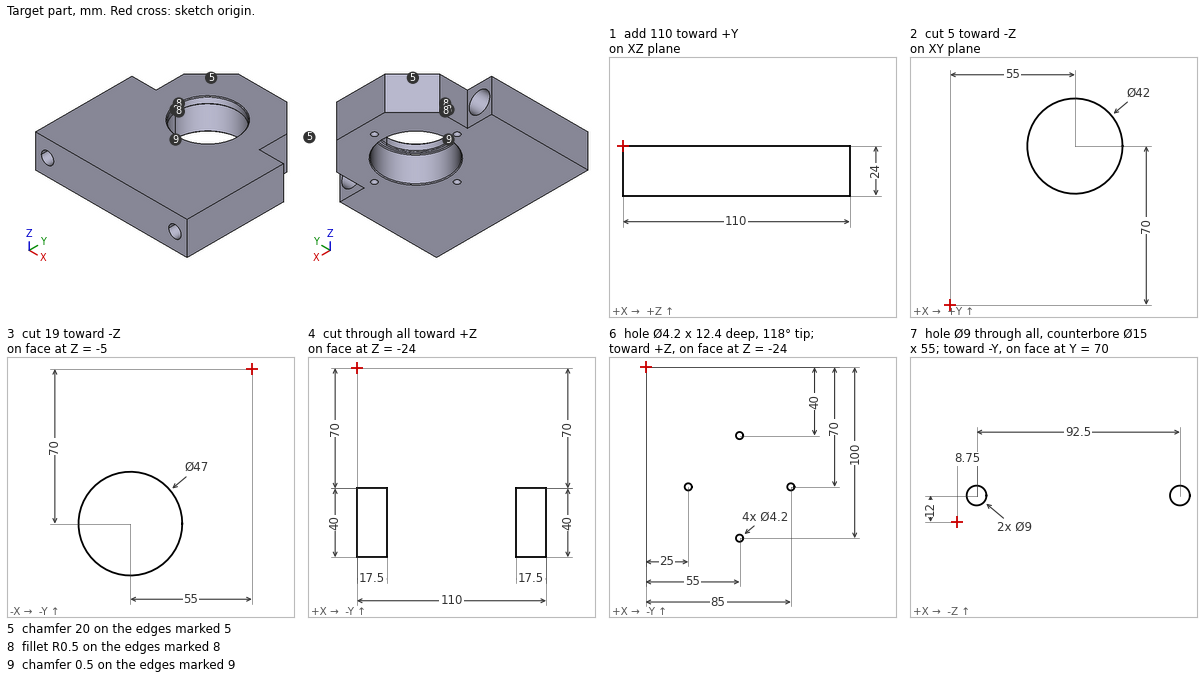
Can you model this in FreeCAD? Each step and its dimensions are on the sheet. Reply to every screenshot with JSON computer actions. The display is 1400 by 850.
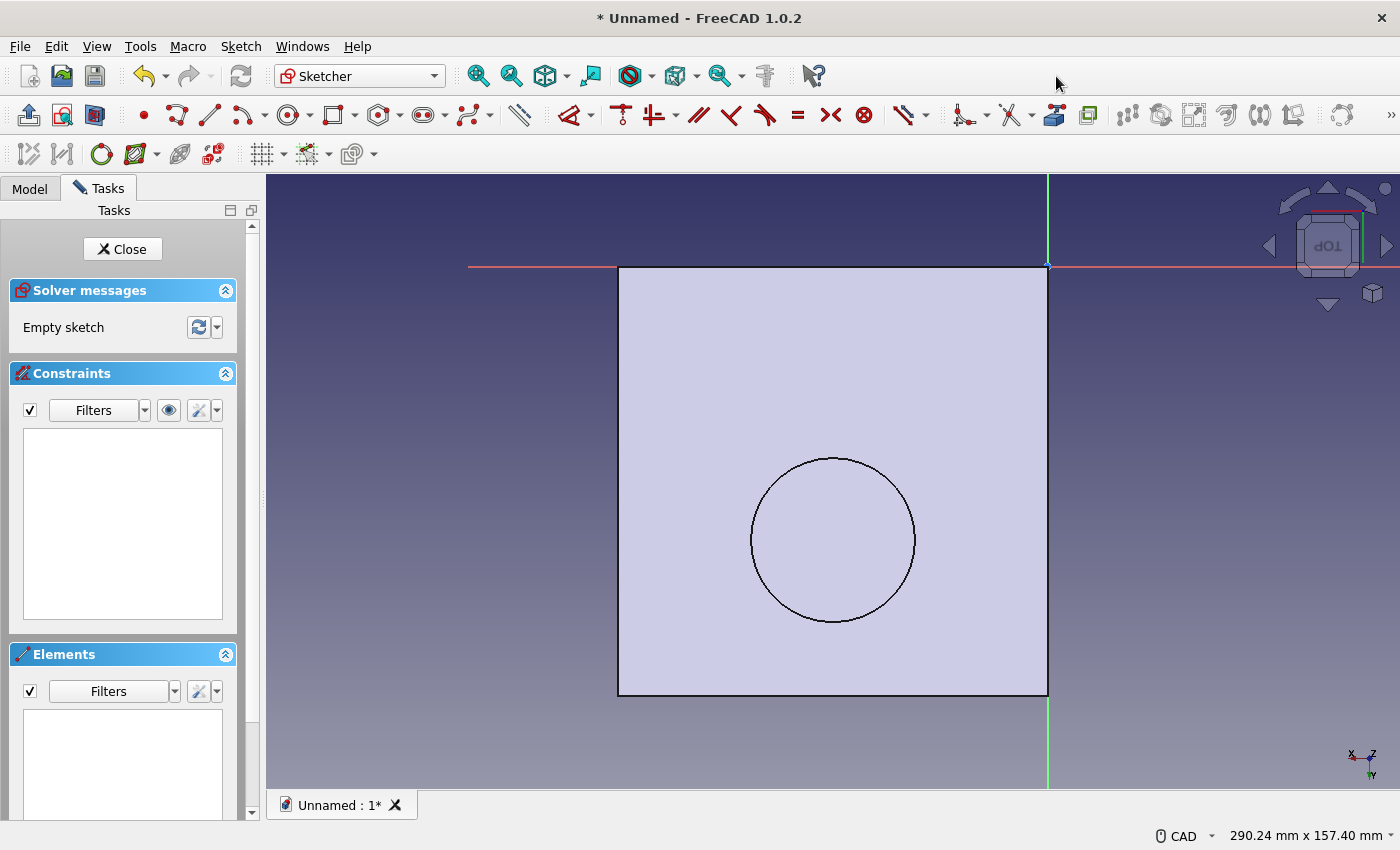
{"action": "left_click", "coordinate": [288, 116]}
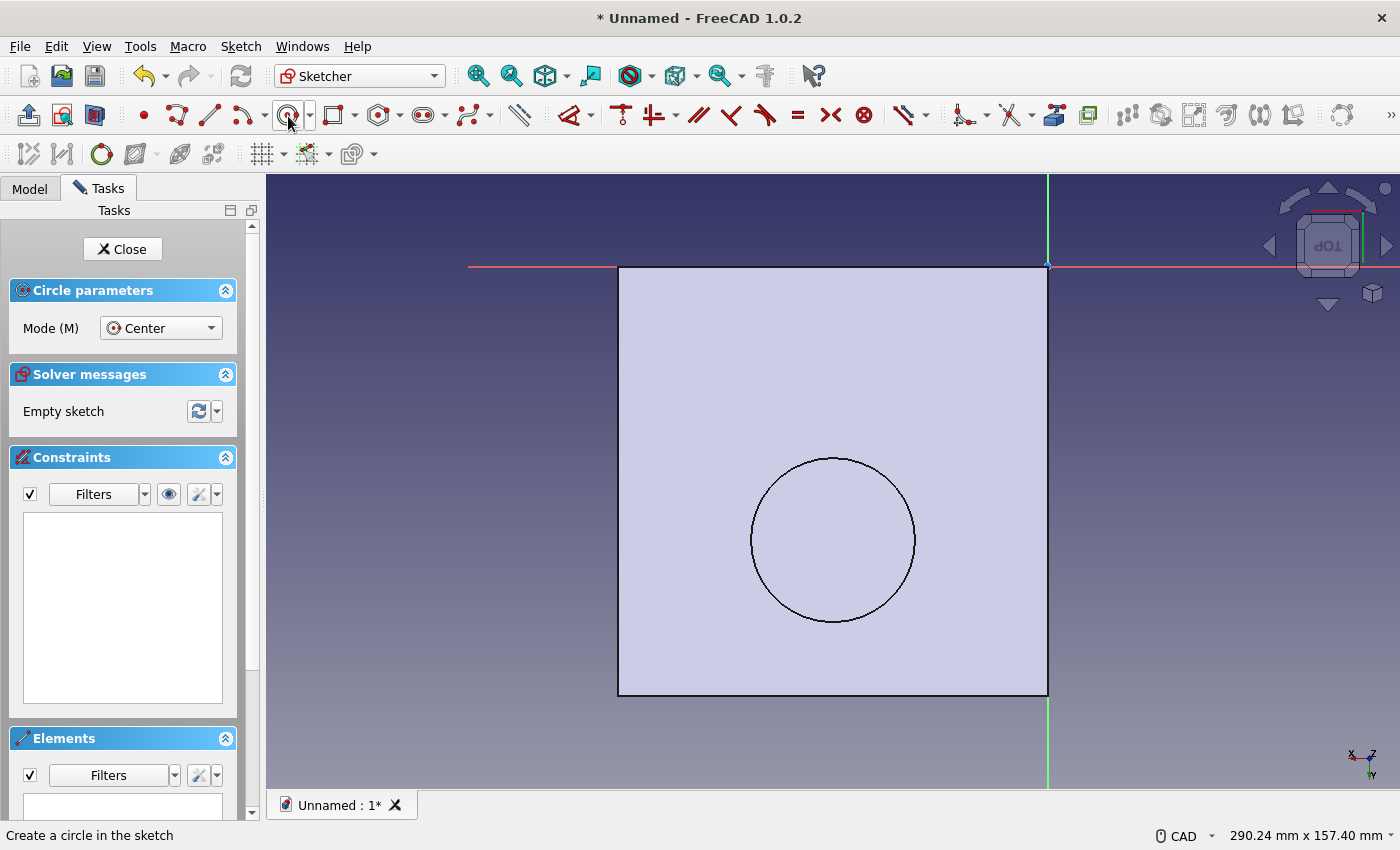
{"action": "left_click", "coordinate": [833, 540]}
{"action": "mouse_move", "coordinate": [898, 475]}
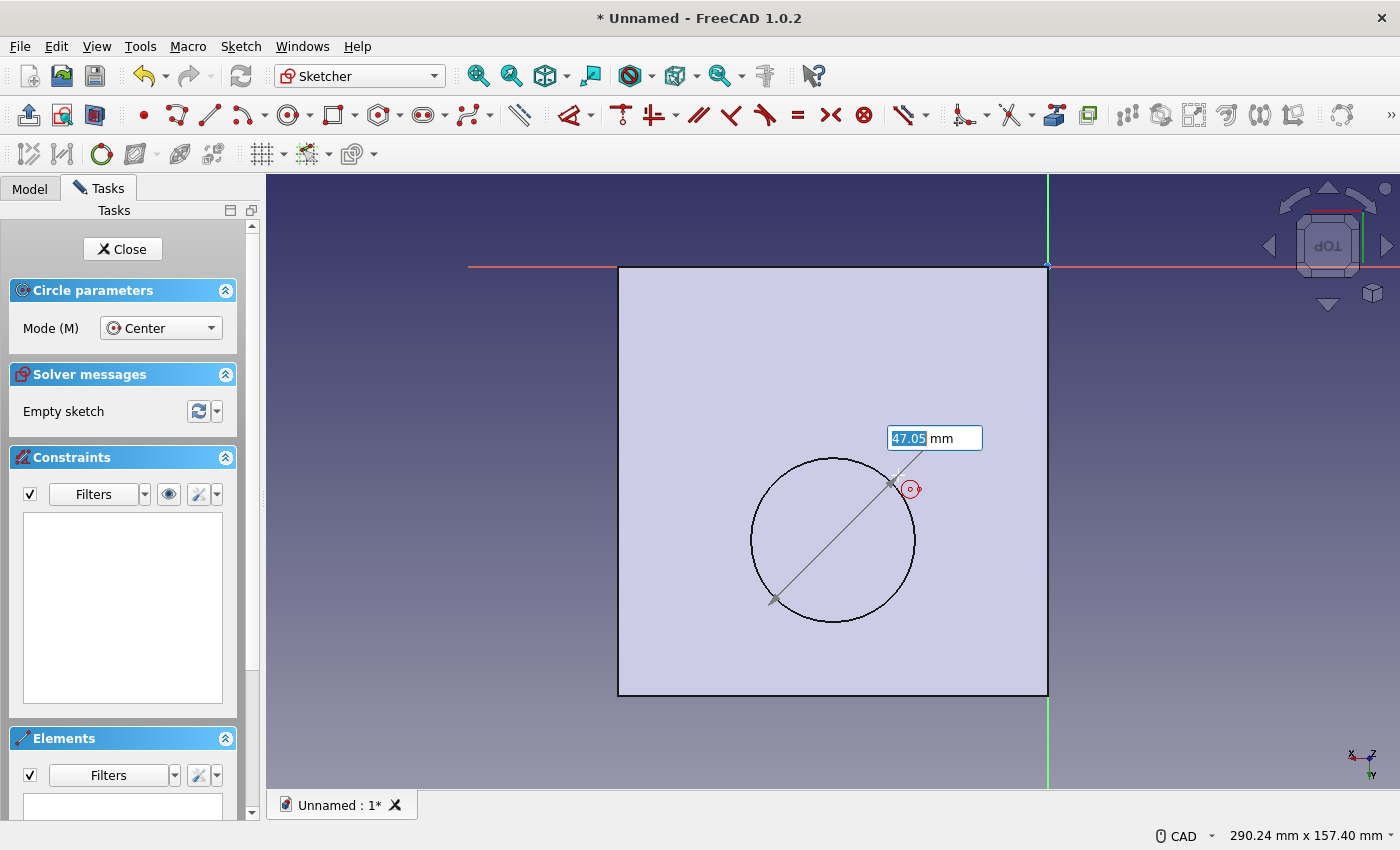
{"action": "type", "text": "47"}
{"action": "key", "text": "Return"}
{"action": "key", "text": "Escape"}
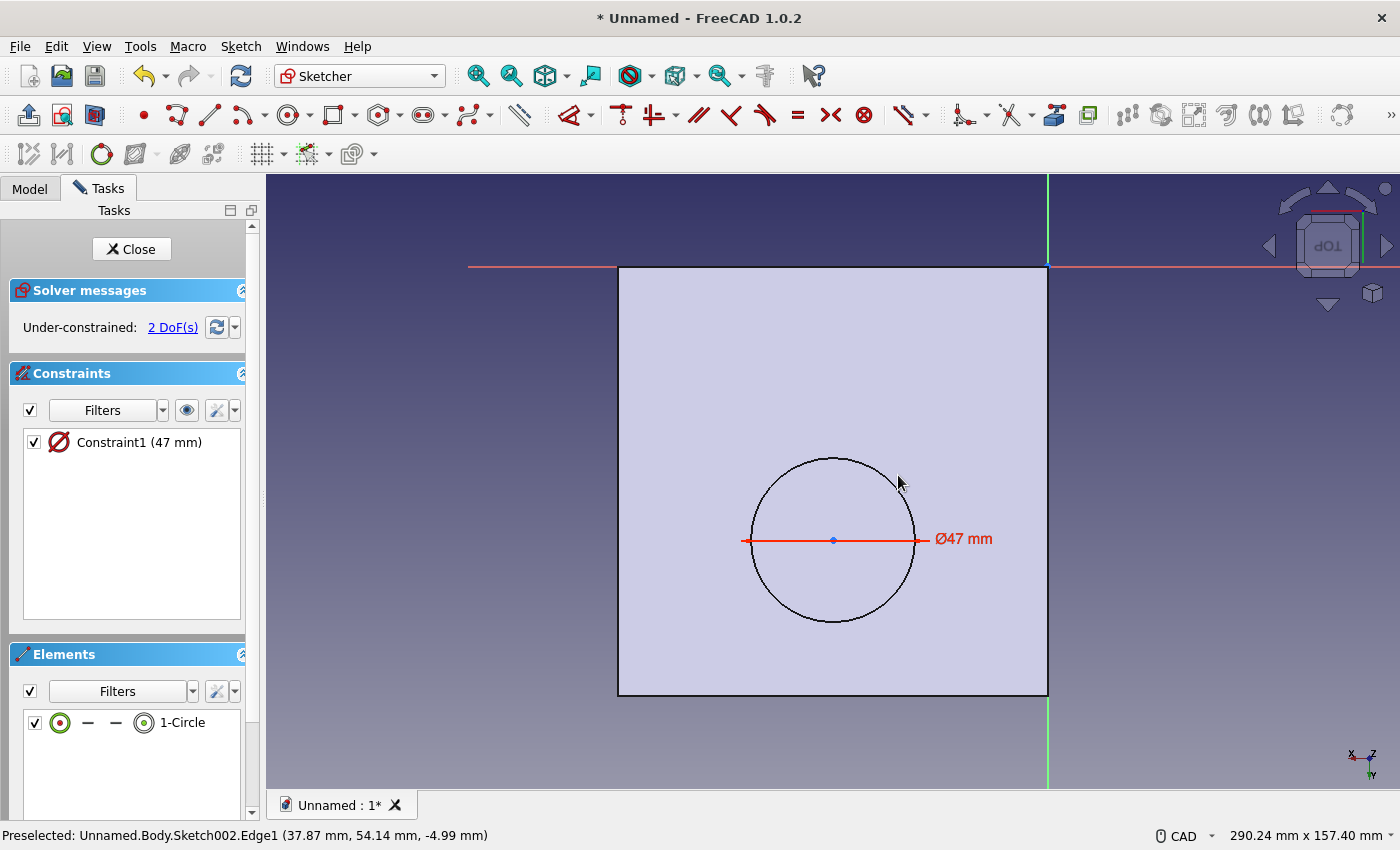
{"action": "left_click", "coordinate": [568, 116]}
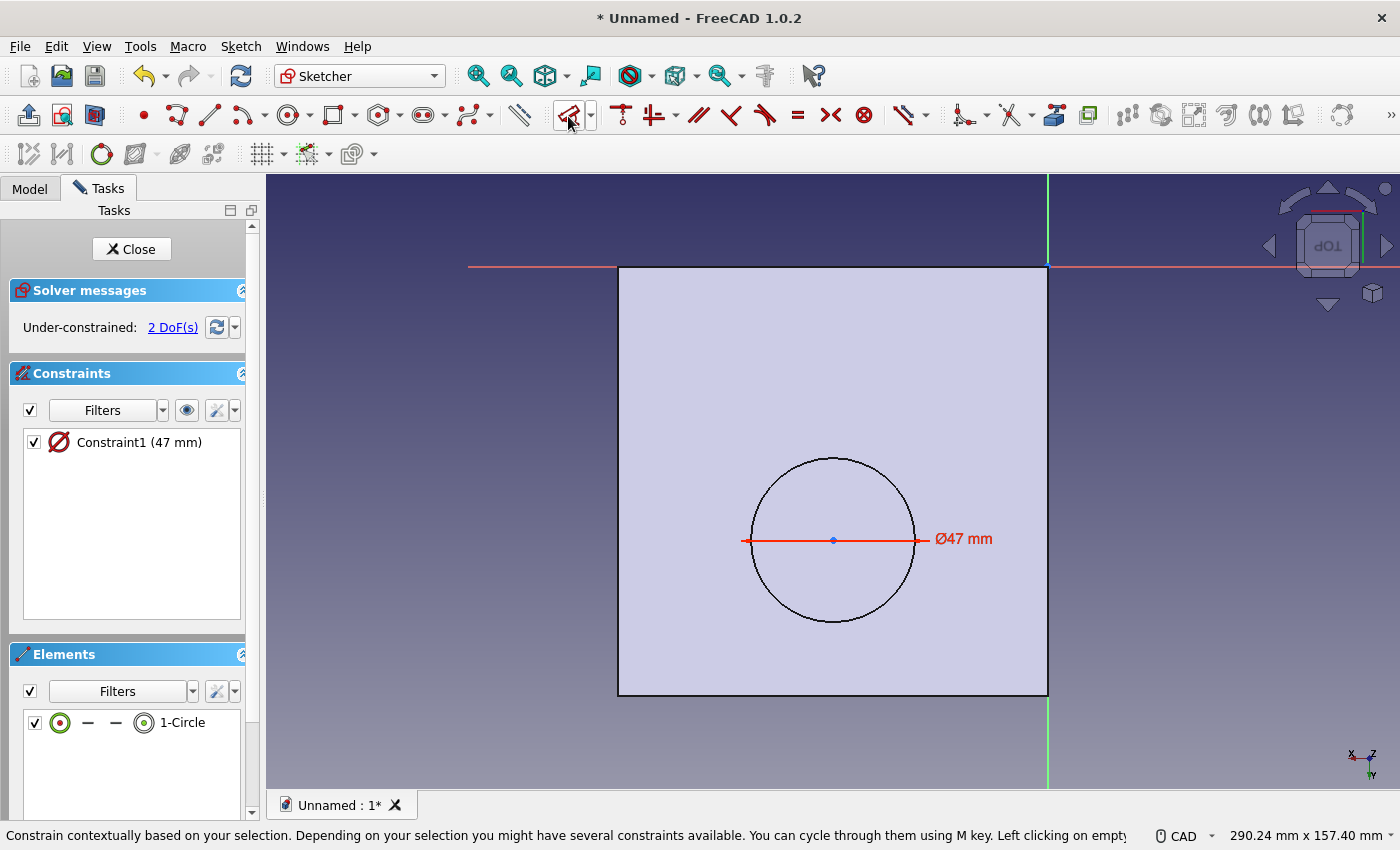
{"action": "left_click", "coordinate": [833, 541]}
{"action": "left_click", "coordinate": [940, 233]}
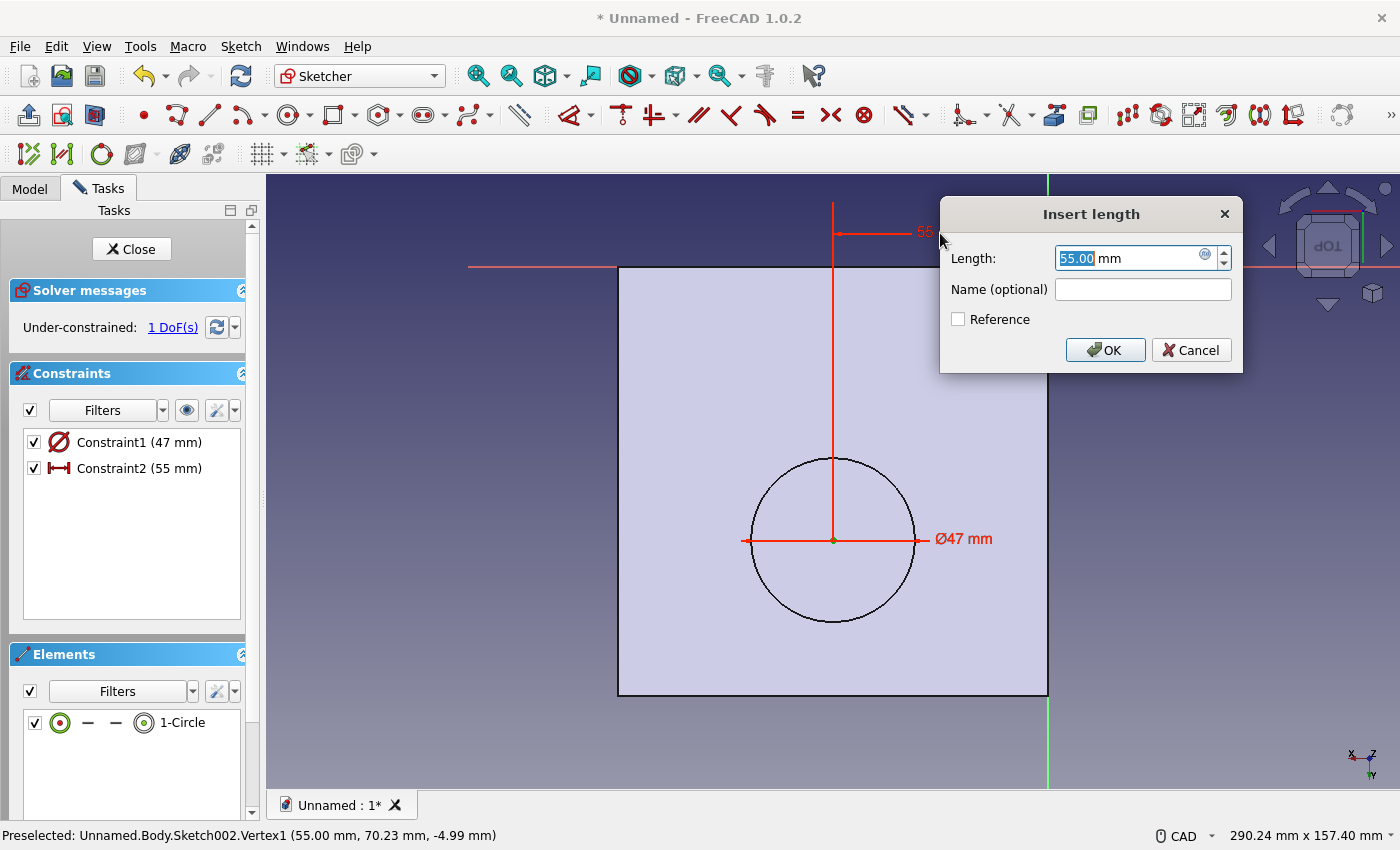
{"action": "type", "text": "55"}
{"action": "key", "text": "Return"}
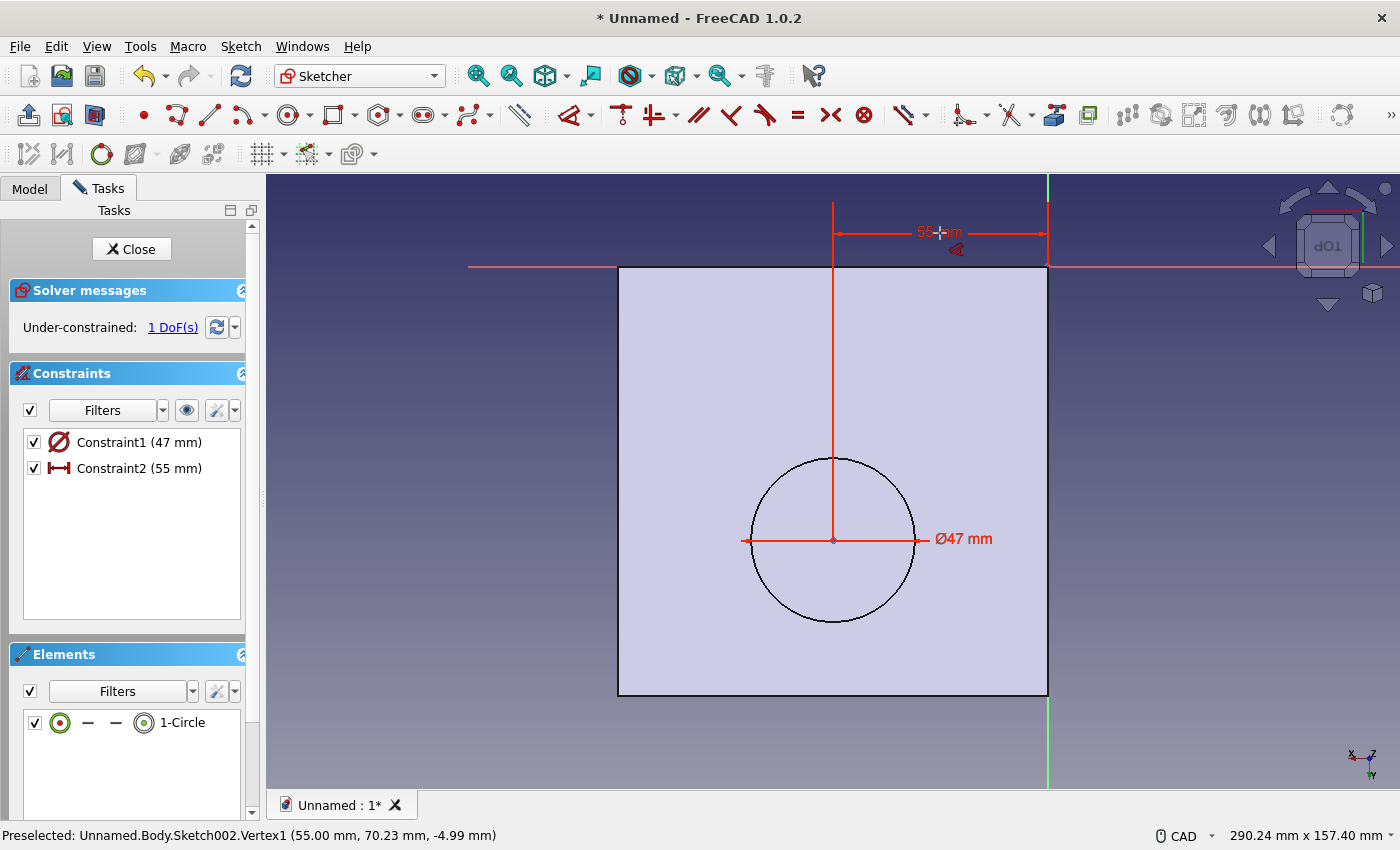
{"action": "left_click", "coordinate": [833, 541]}
{"action": "left_click", "coordinate": [1082, 404]}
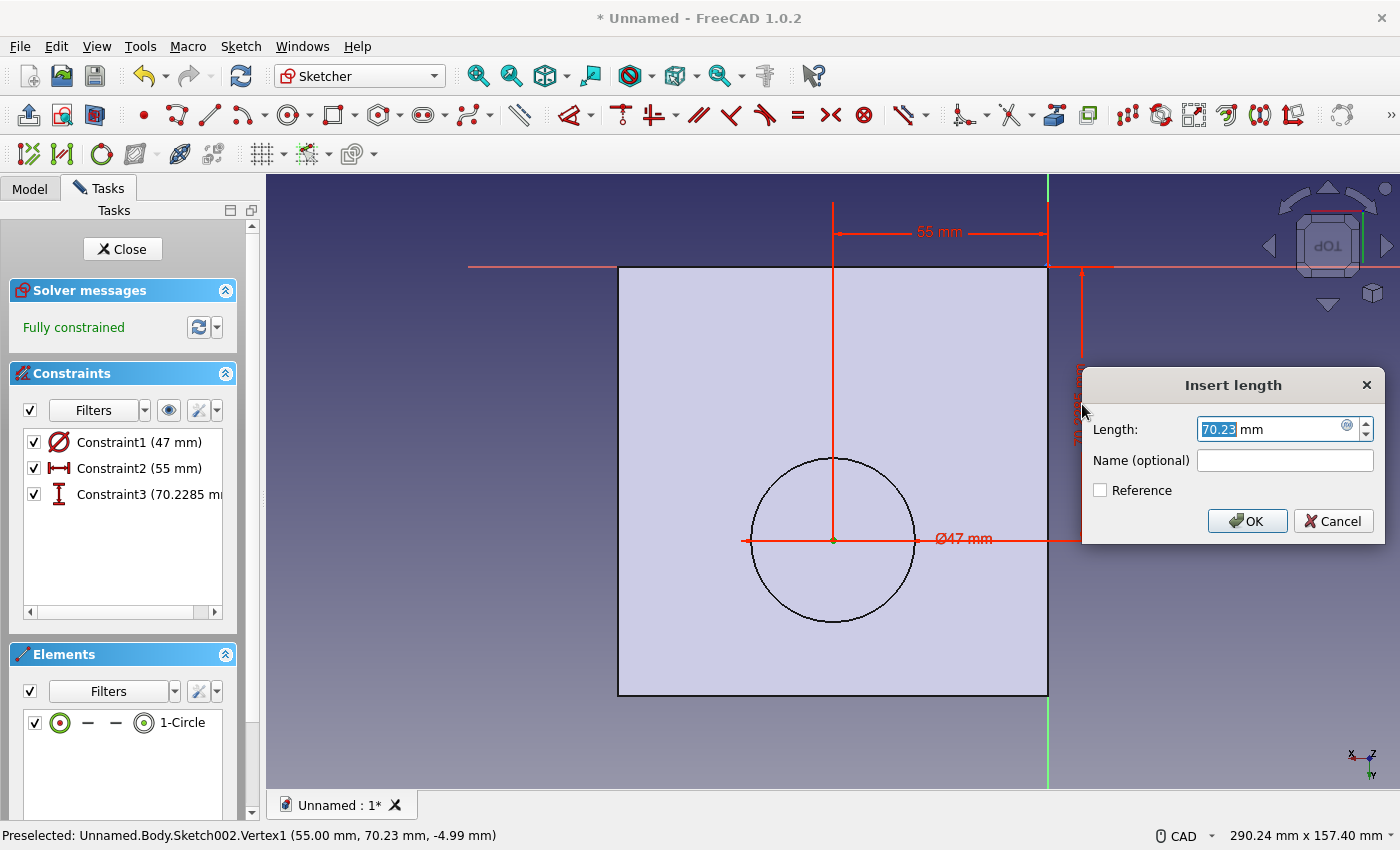
{"action": "type", "text": "70"}
{"action": "key", "text": "Return"}
{"action": "key", "text": "Escape"}